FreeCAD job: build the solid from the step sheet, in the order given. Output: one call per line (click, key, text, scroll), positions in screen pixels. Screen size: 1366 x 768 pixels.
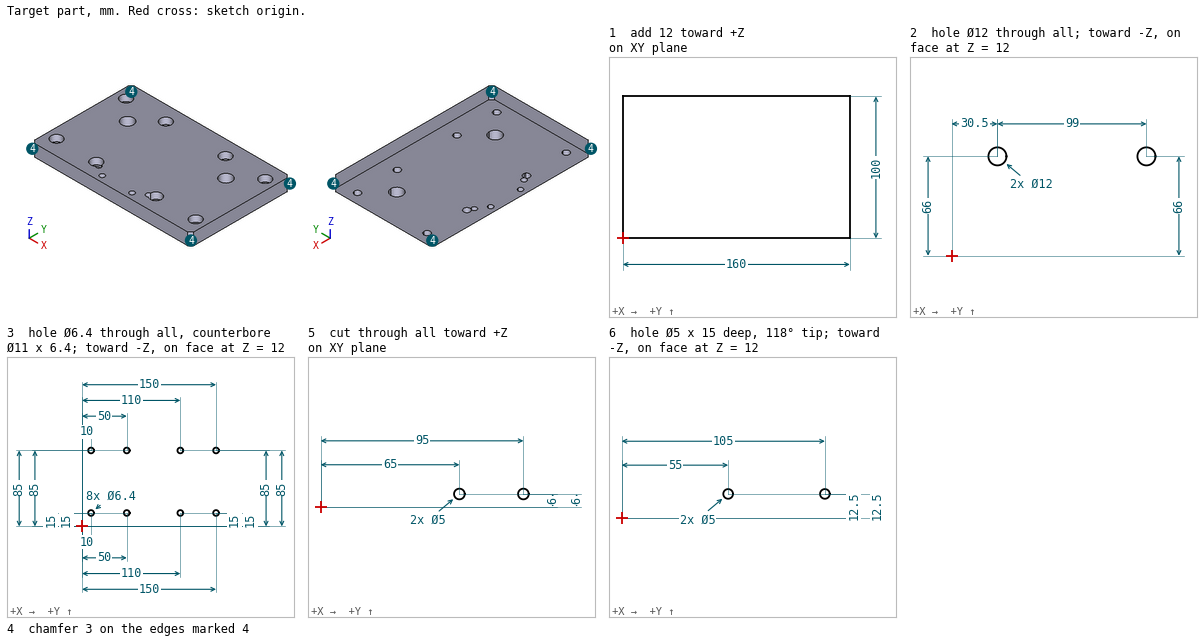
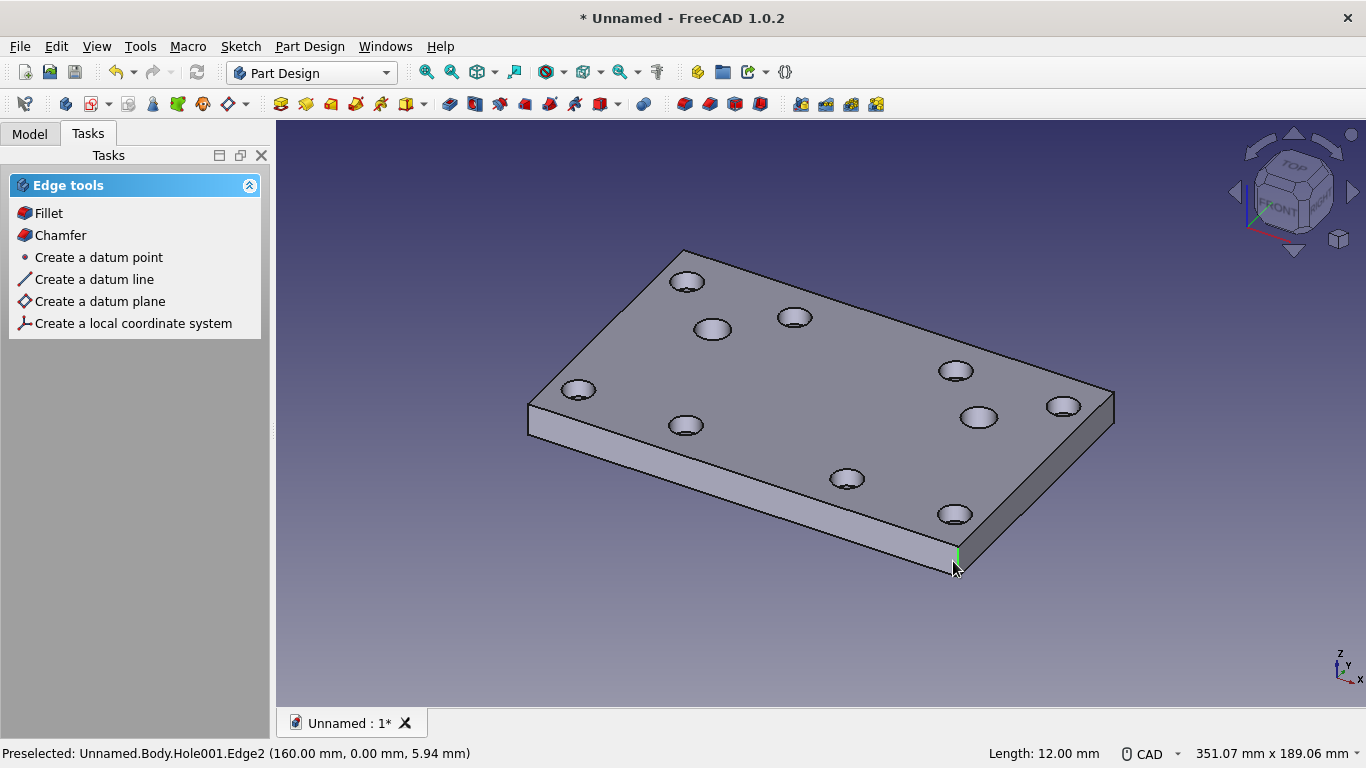
key(0)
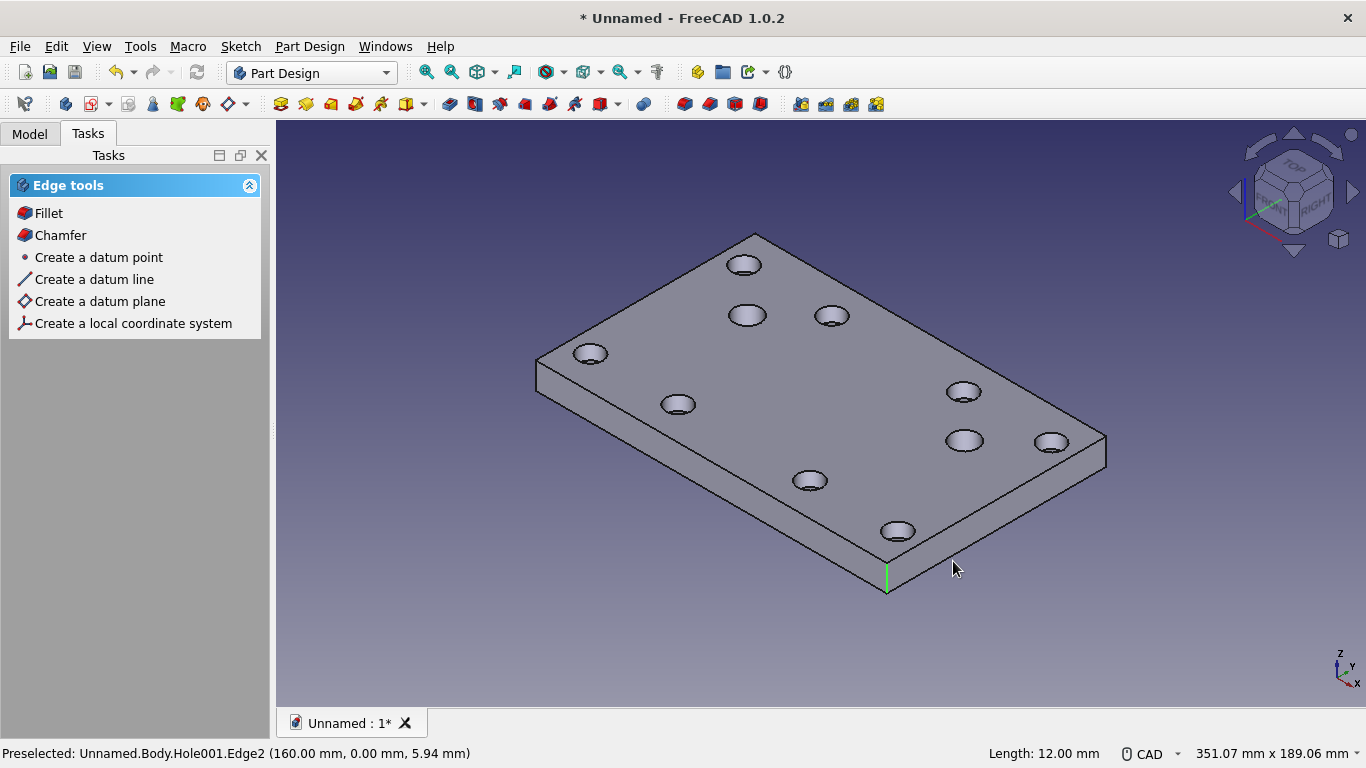
key(2)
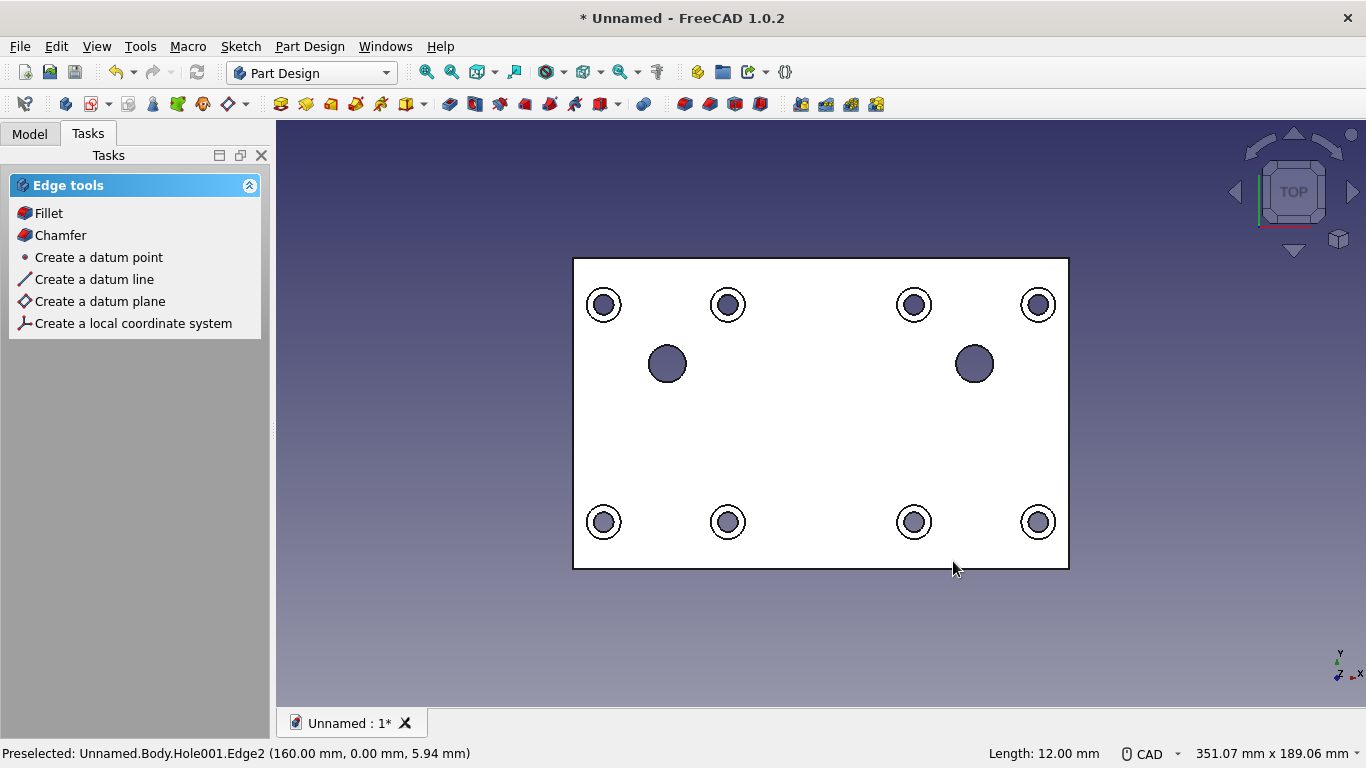
key(1)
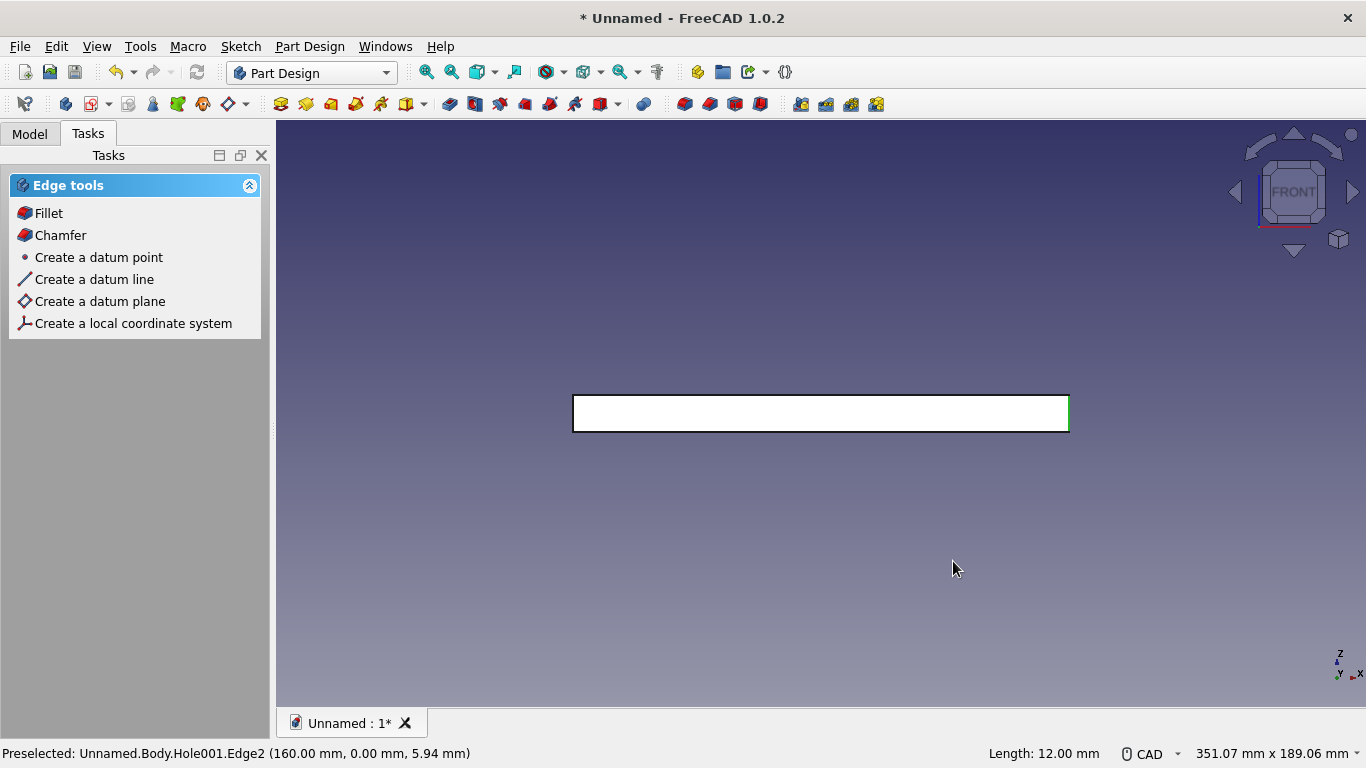
click(573, 412, ctrl)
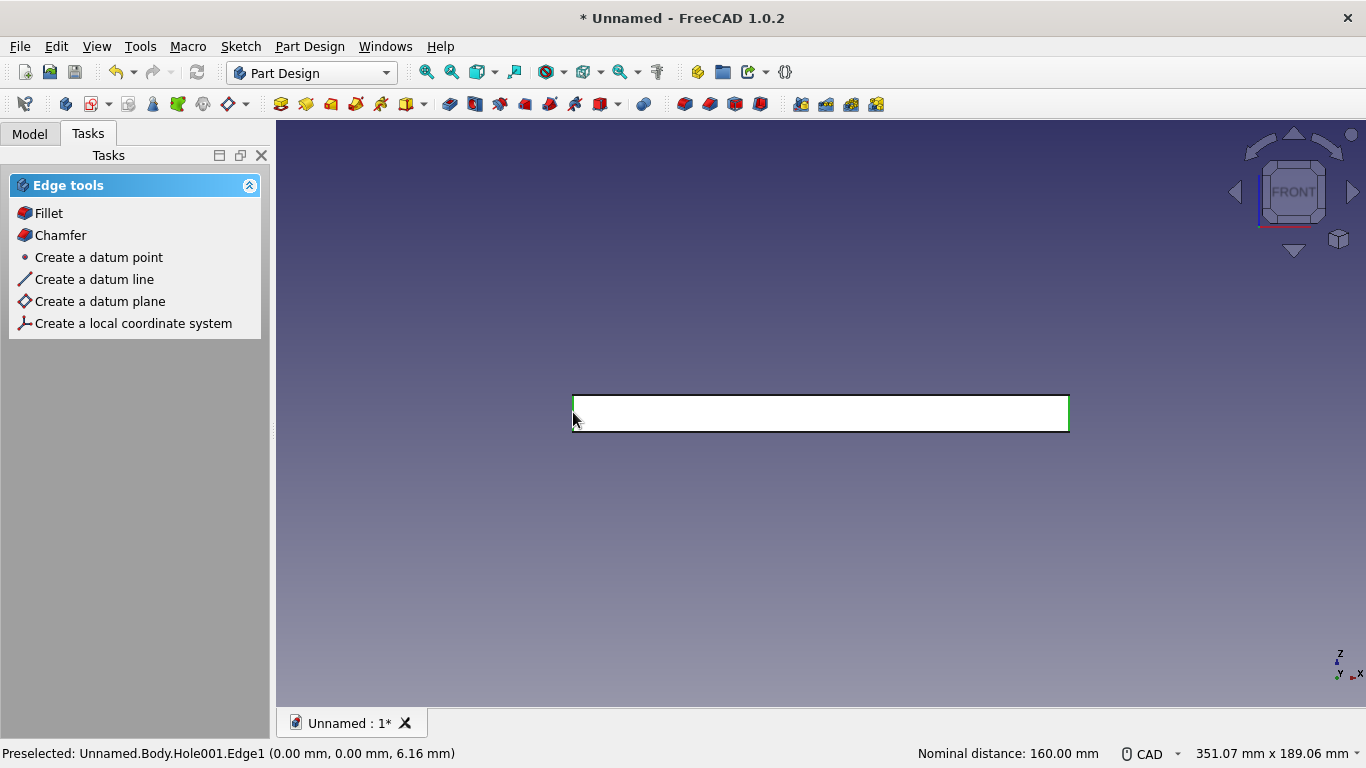
key(3)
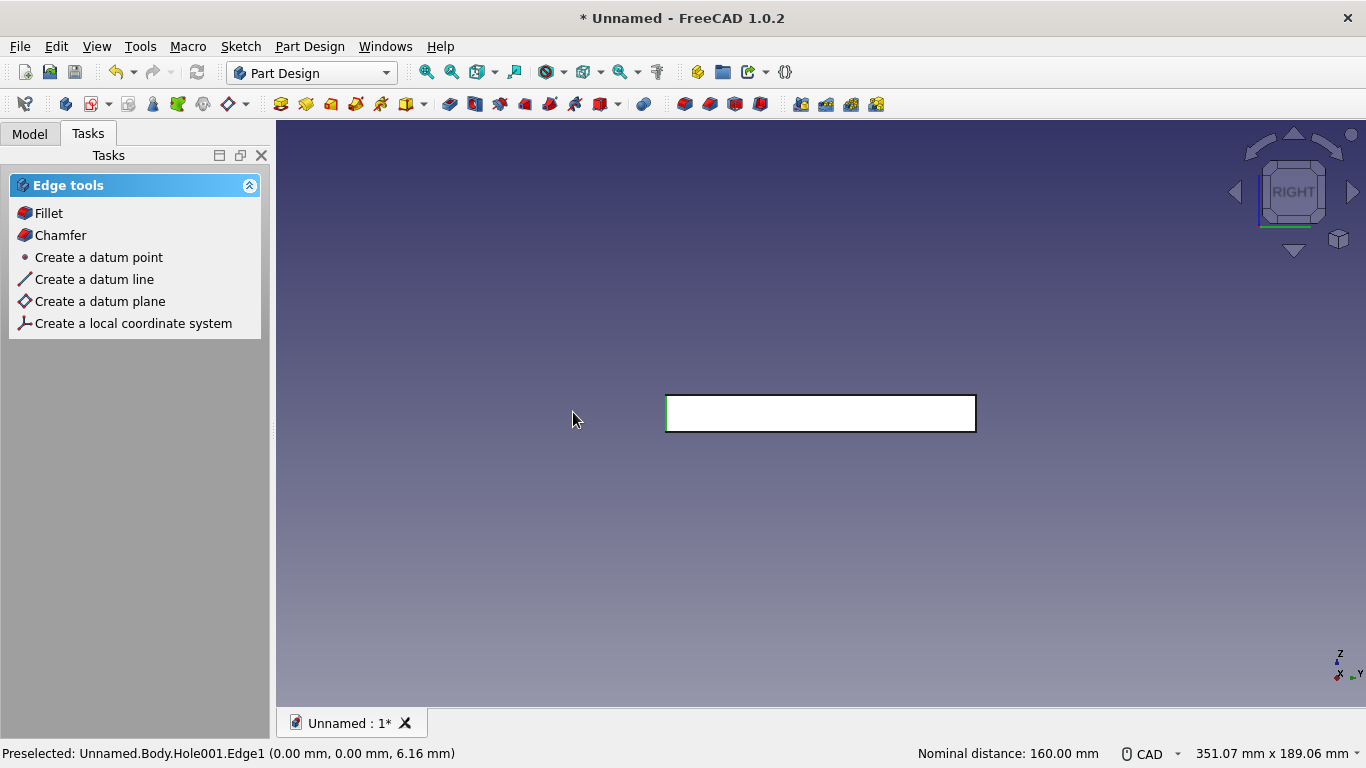
key(v)
key(f)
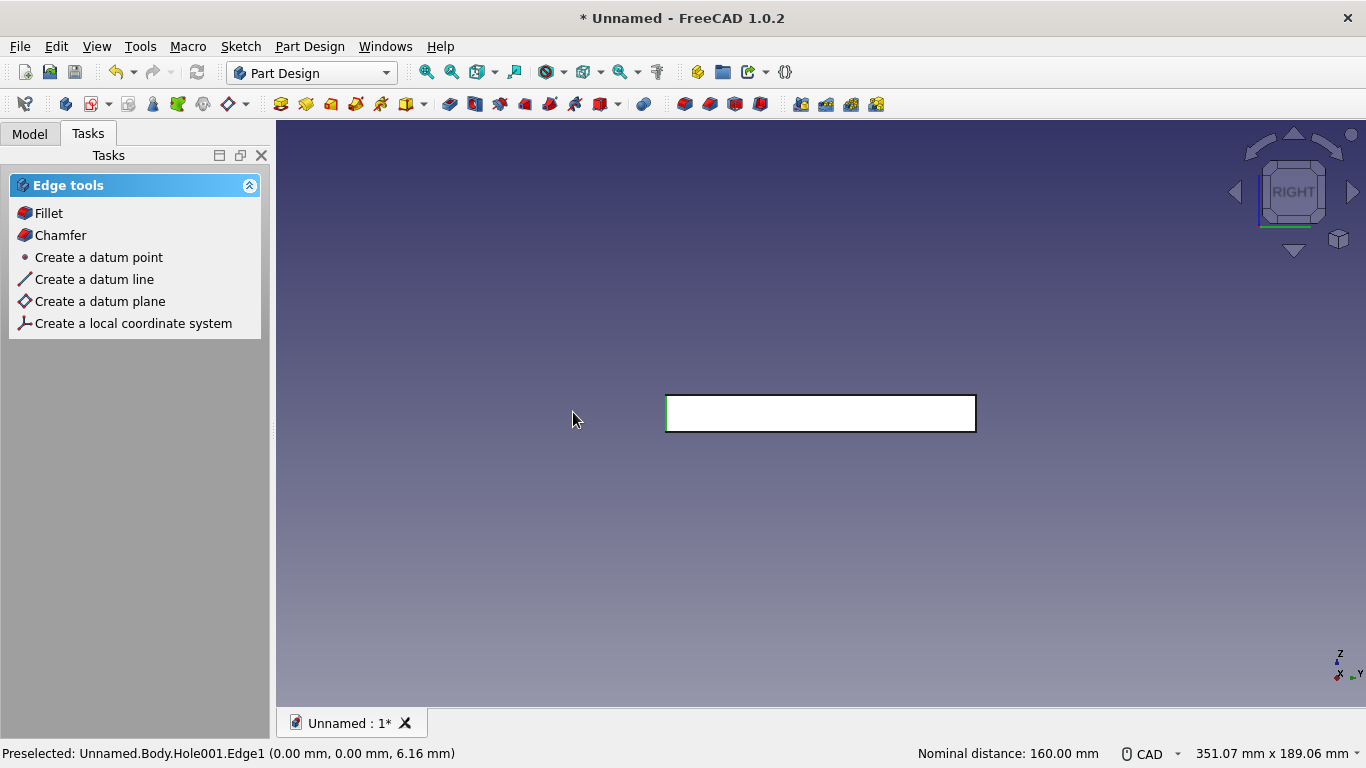
click(976, 412, ctrl)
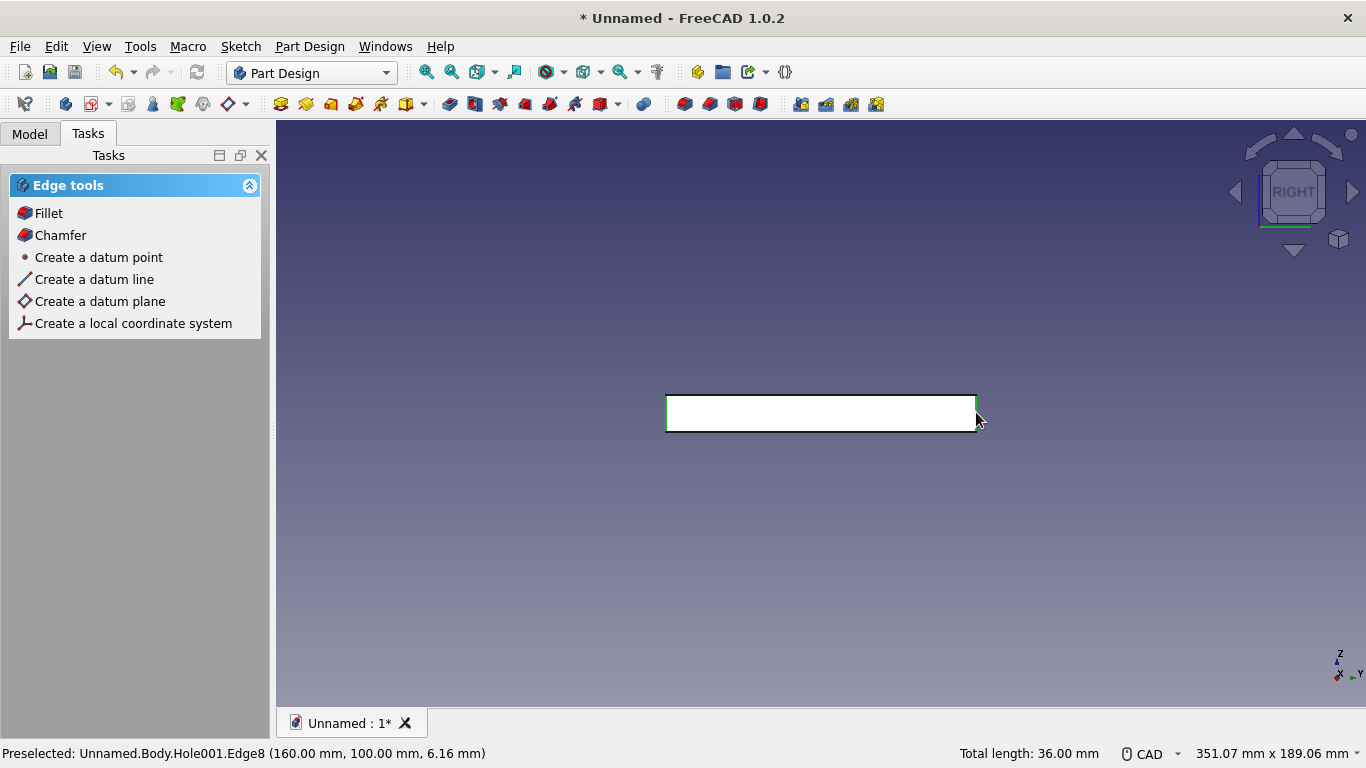
key(5)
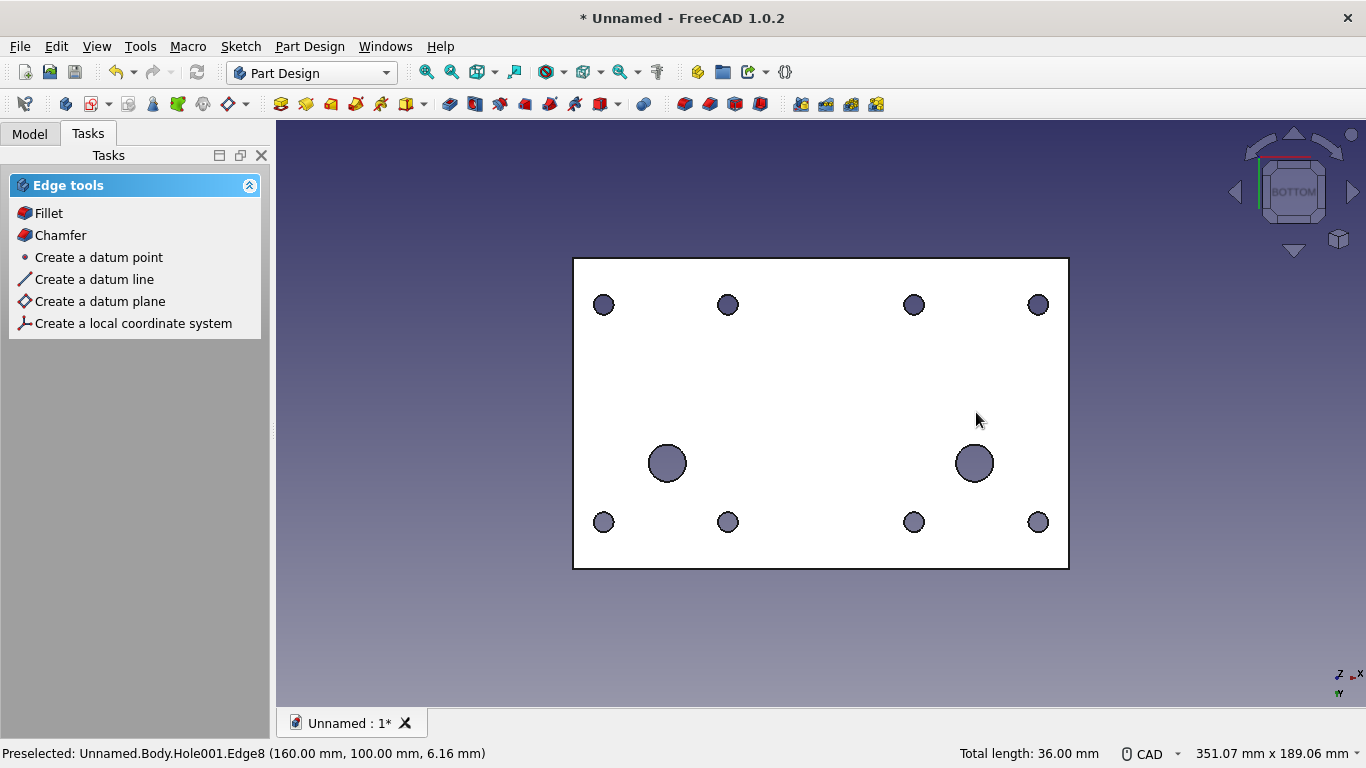
key(4)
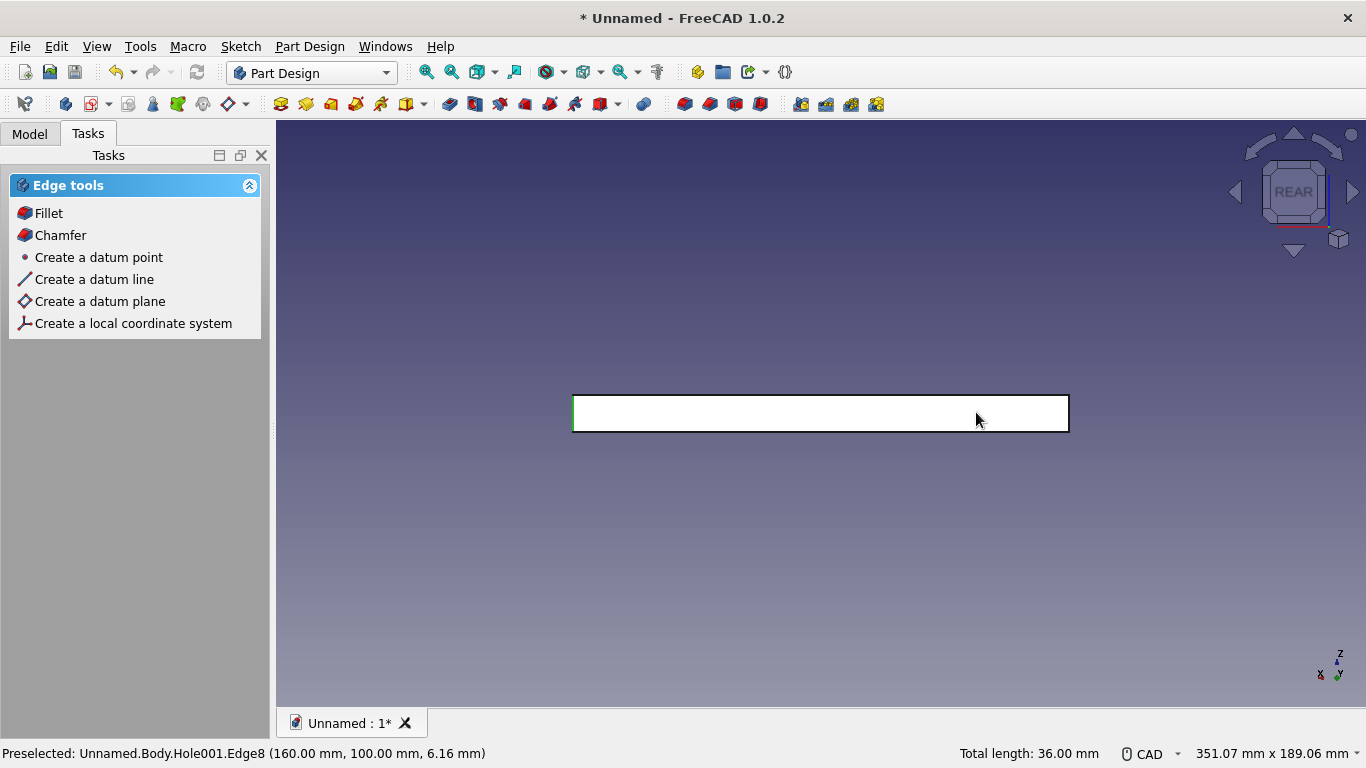
click(1069, 412, ctrl)